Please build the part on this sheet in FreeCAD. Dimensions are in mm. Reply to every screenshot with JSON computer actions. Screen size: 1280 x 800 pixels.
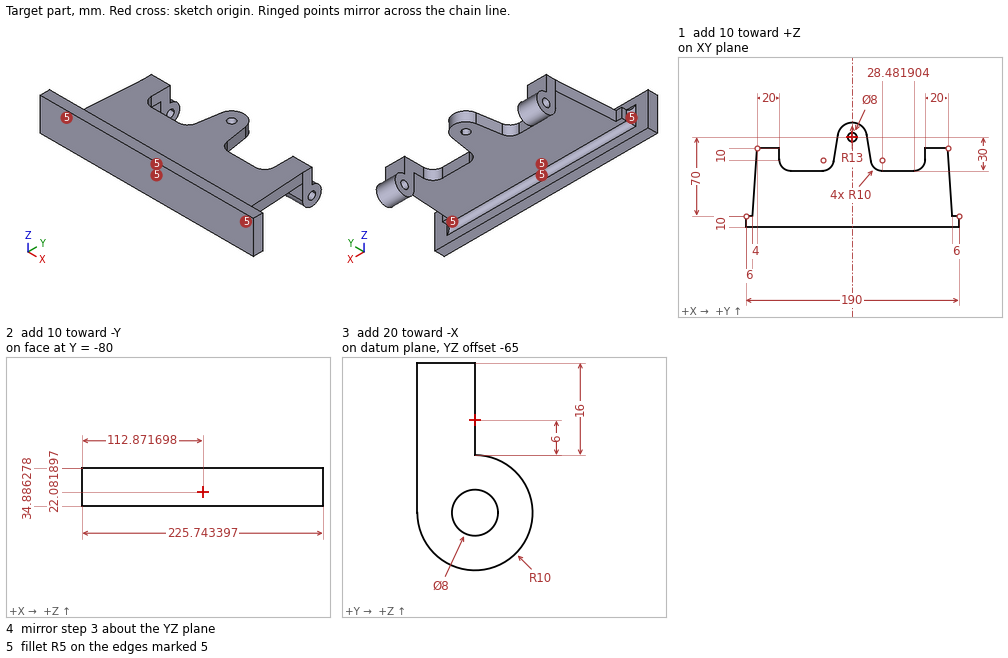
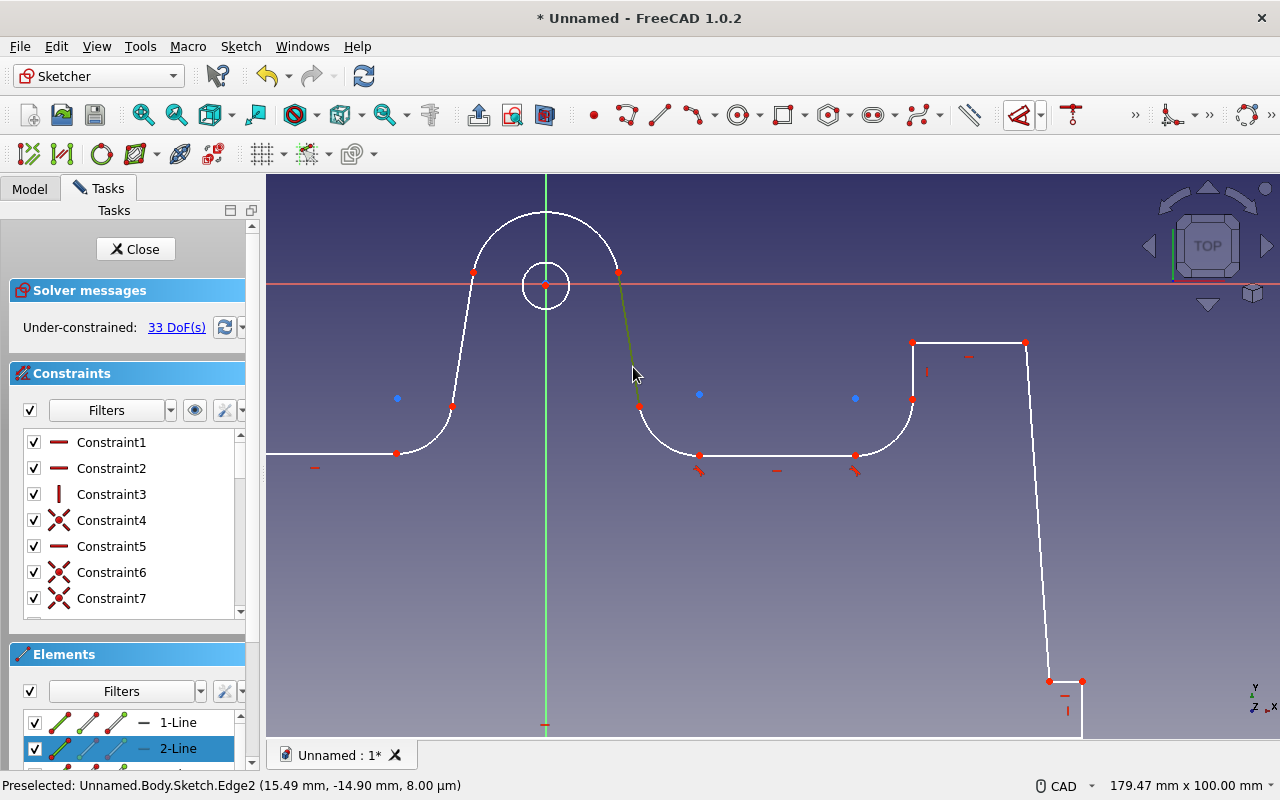
{"action": "left_click", "coordinate": [649, 430]}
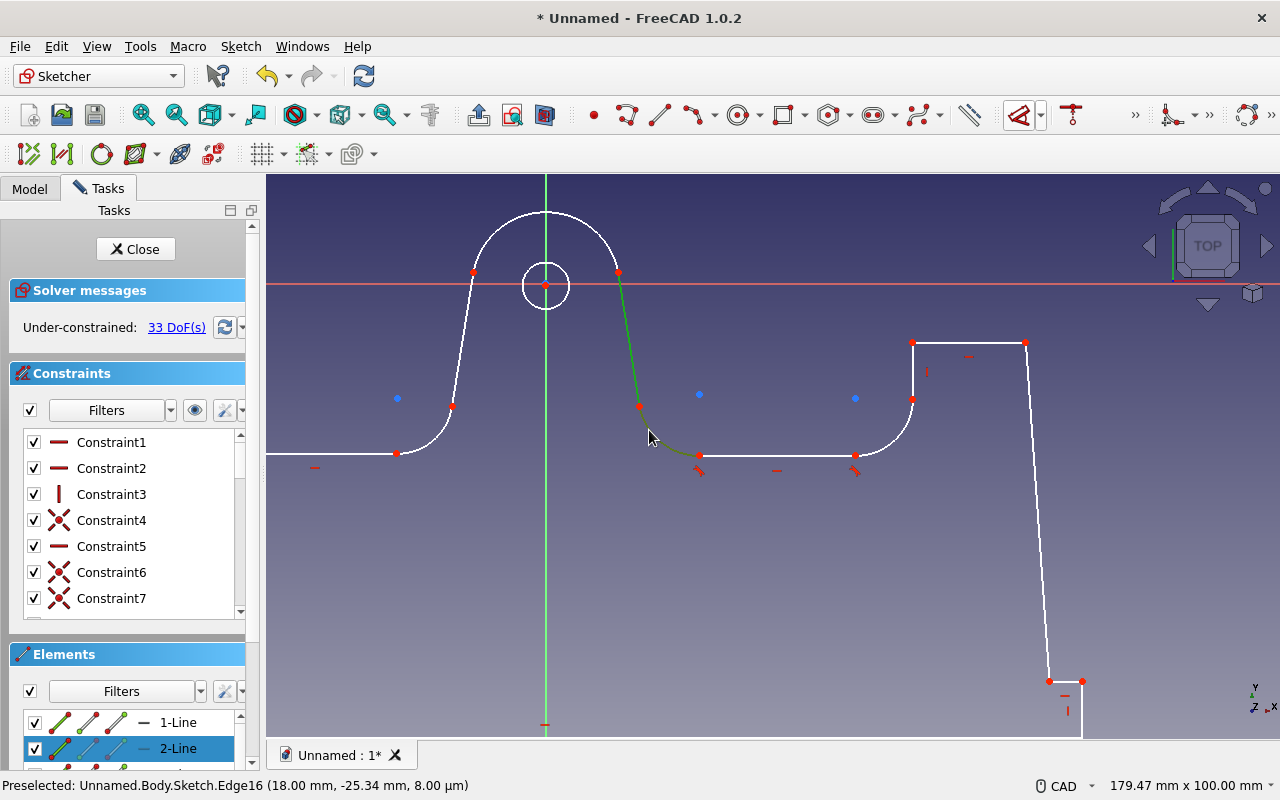
{"action": "key", "text": "t"}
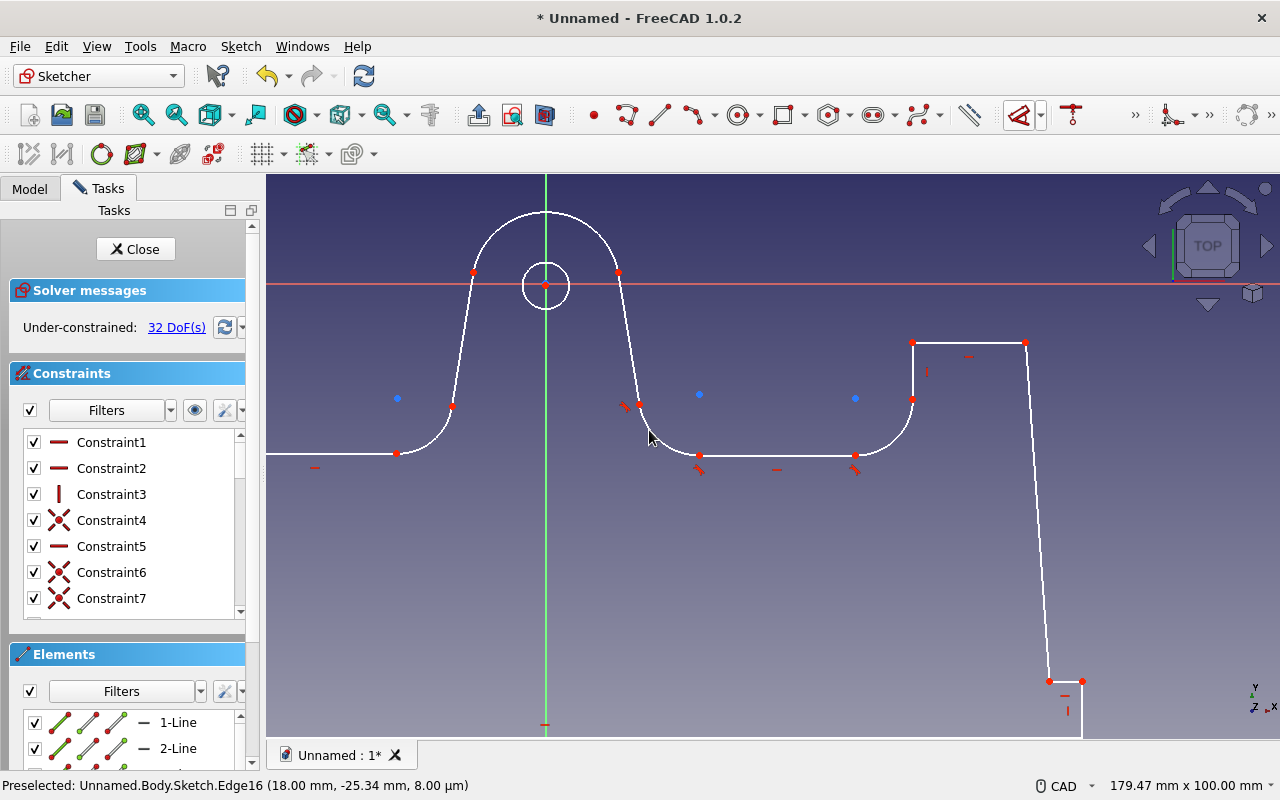
{"action": "left_click", "coordinate": [633, 365]}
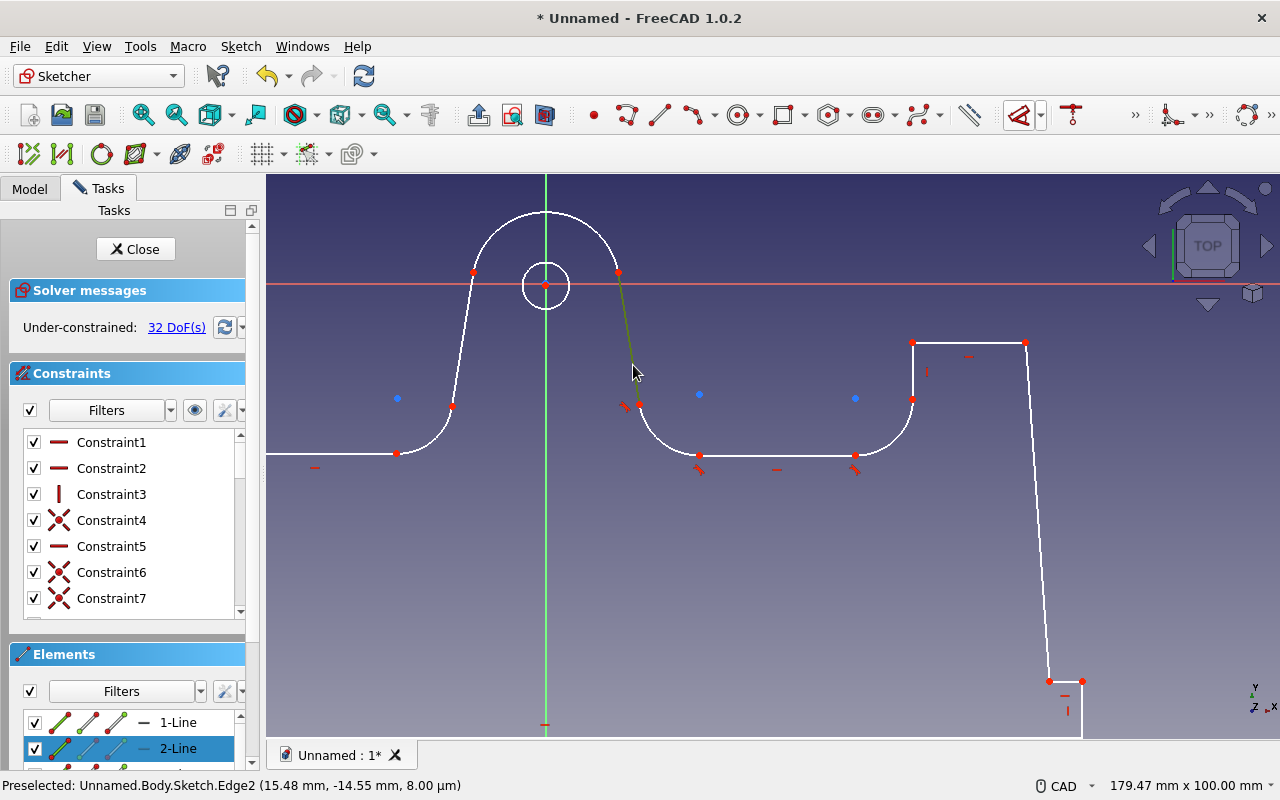
{"action": "left_click", "coordinate": [585, 223]}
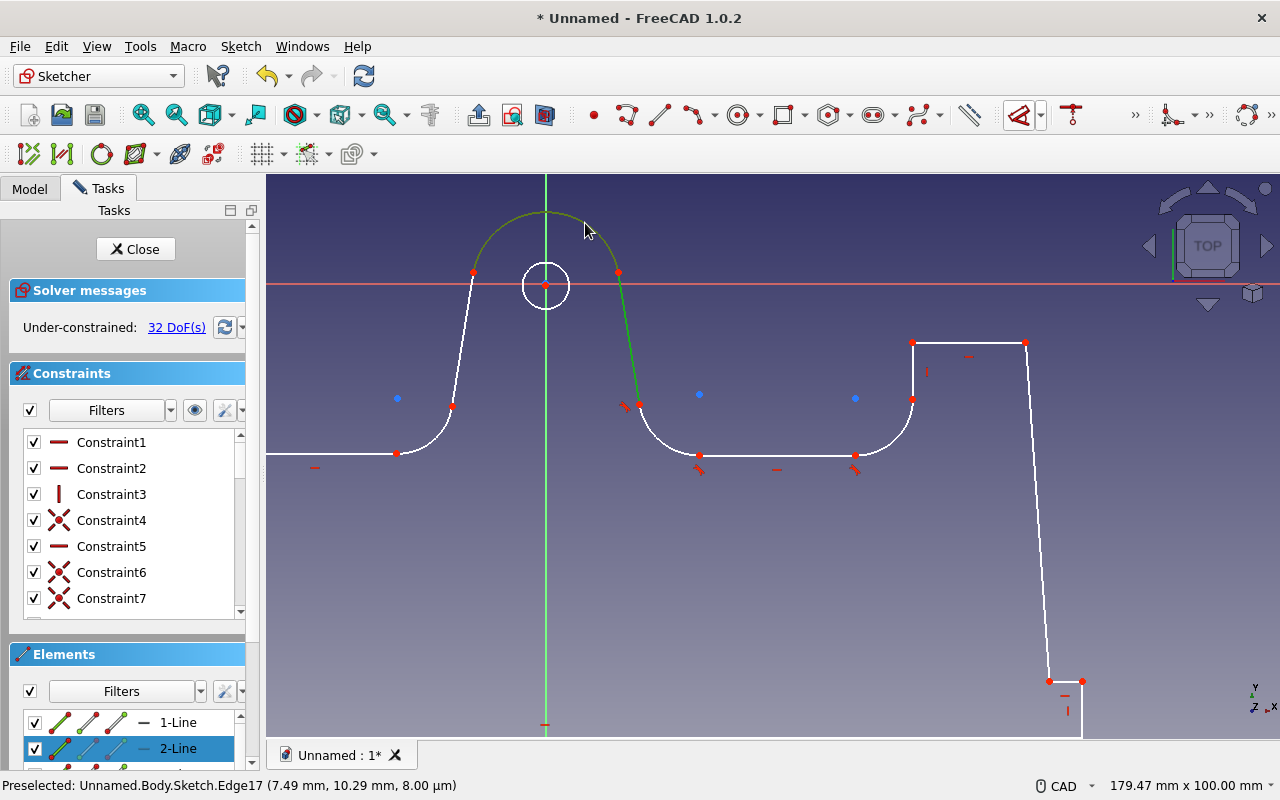
{"action": "key", "text": "t"}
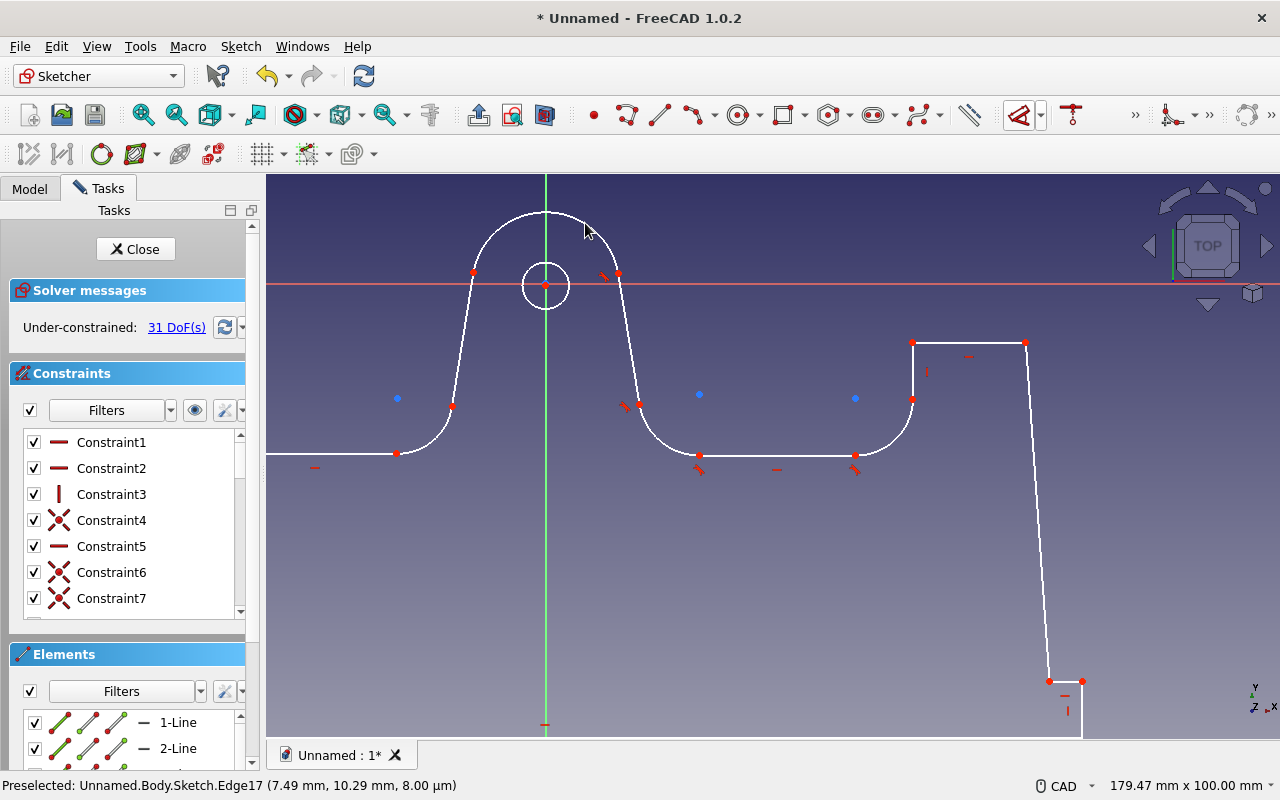
{"action": "left_click", "coordinate": [467, 313]}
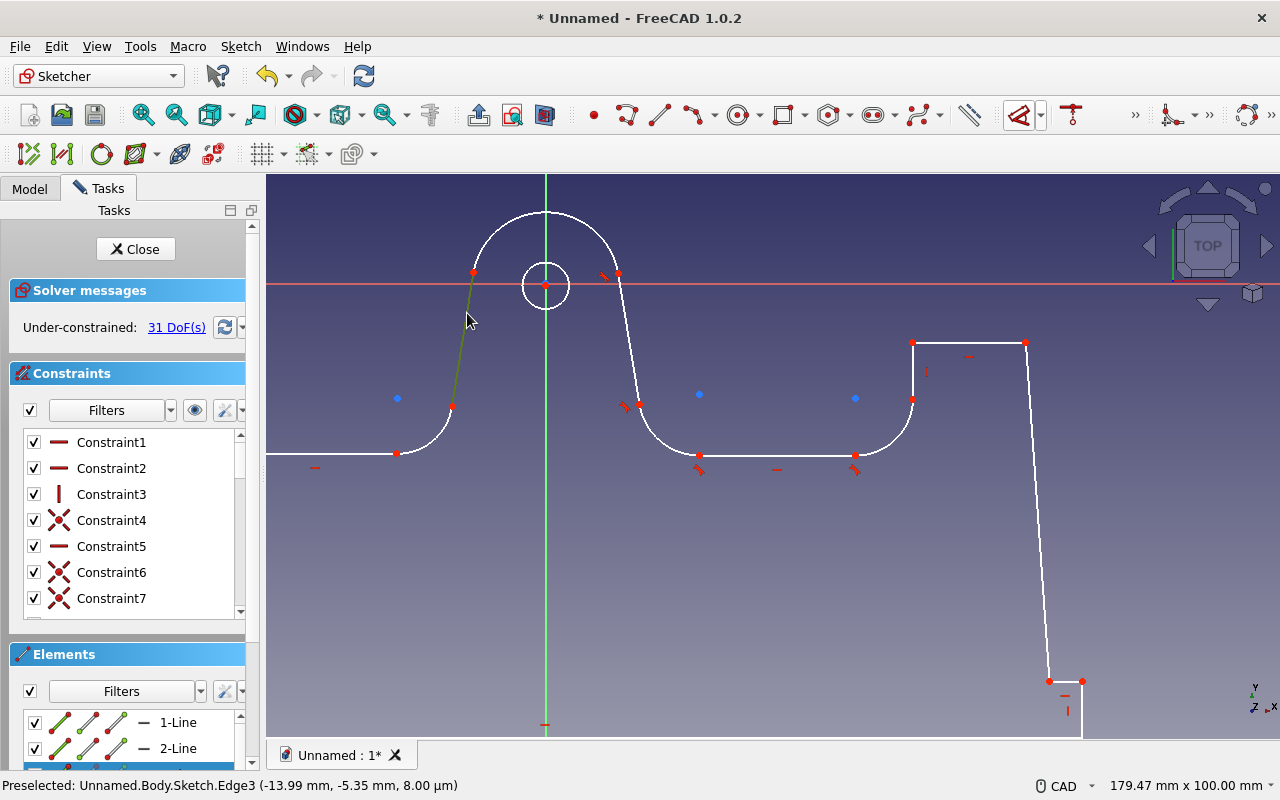
{"action": "left_click", "coordinate": [585, 224]}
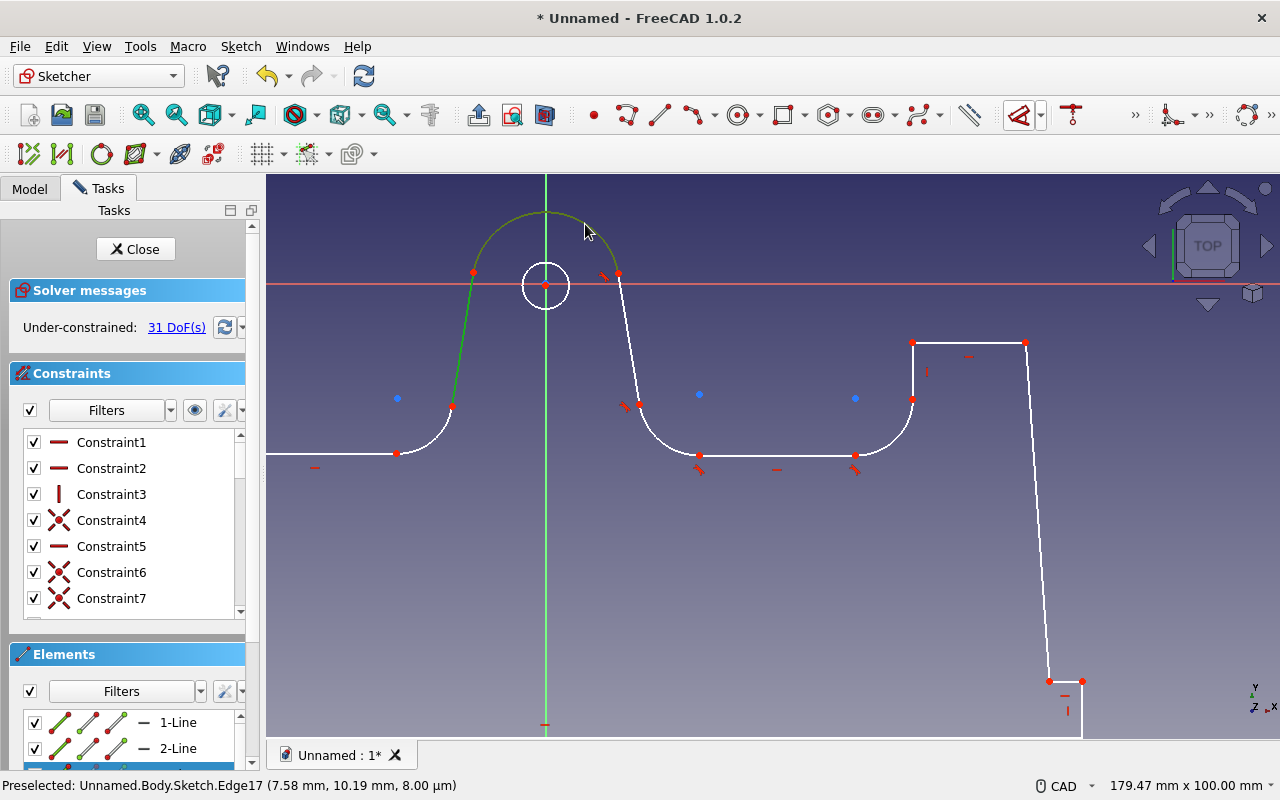
{"action": "key", "text": "t"}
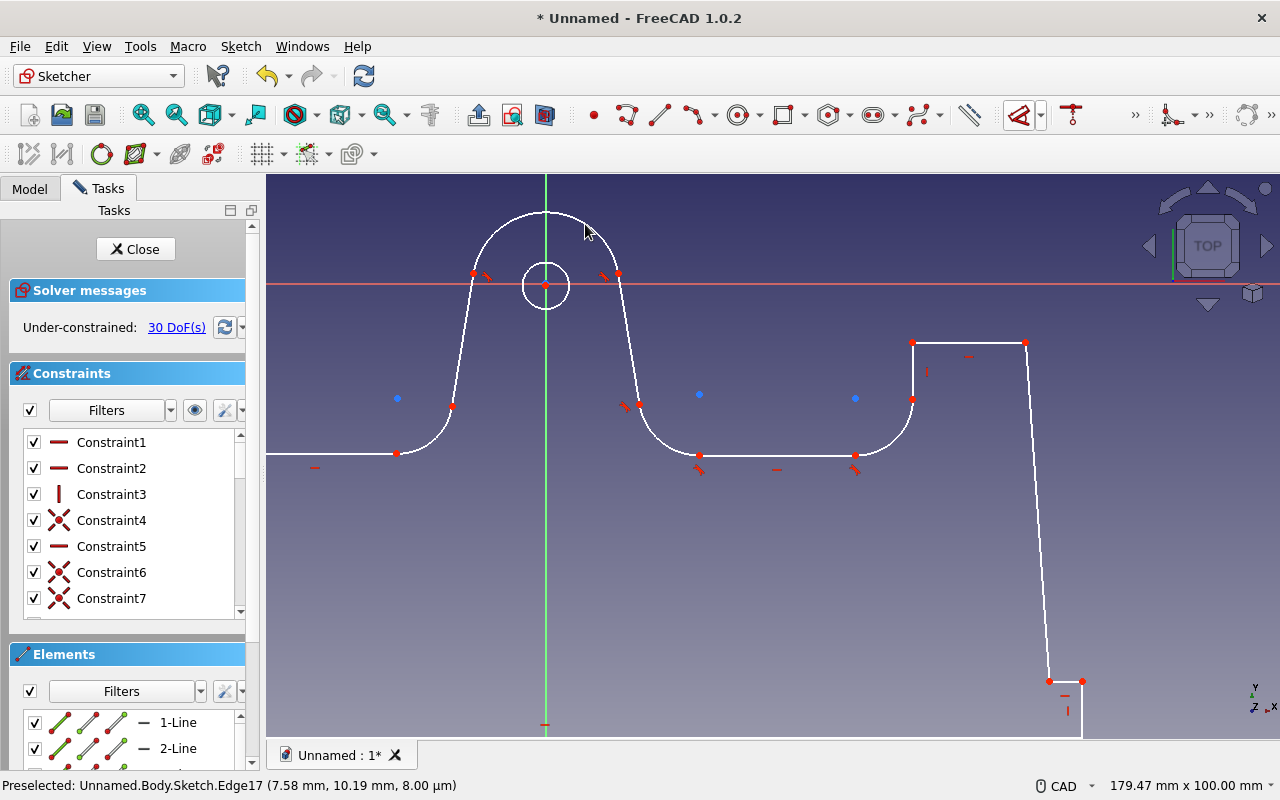
{"action": "left_click", "coordinate": [467, 314]}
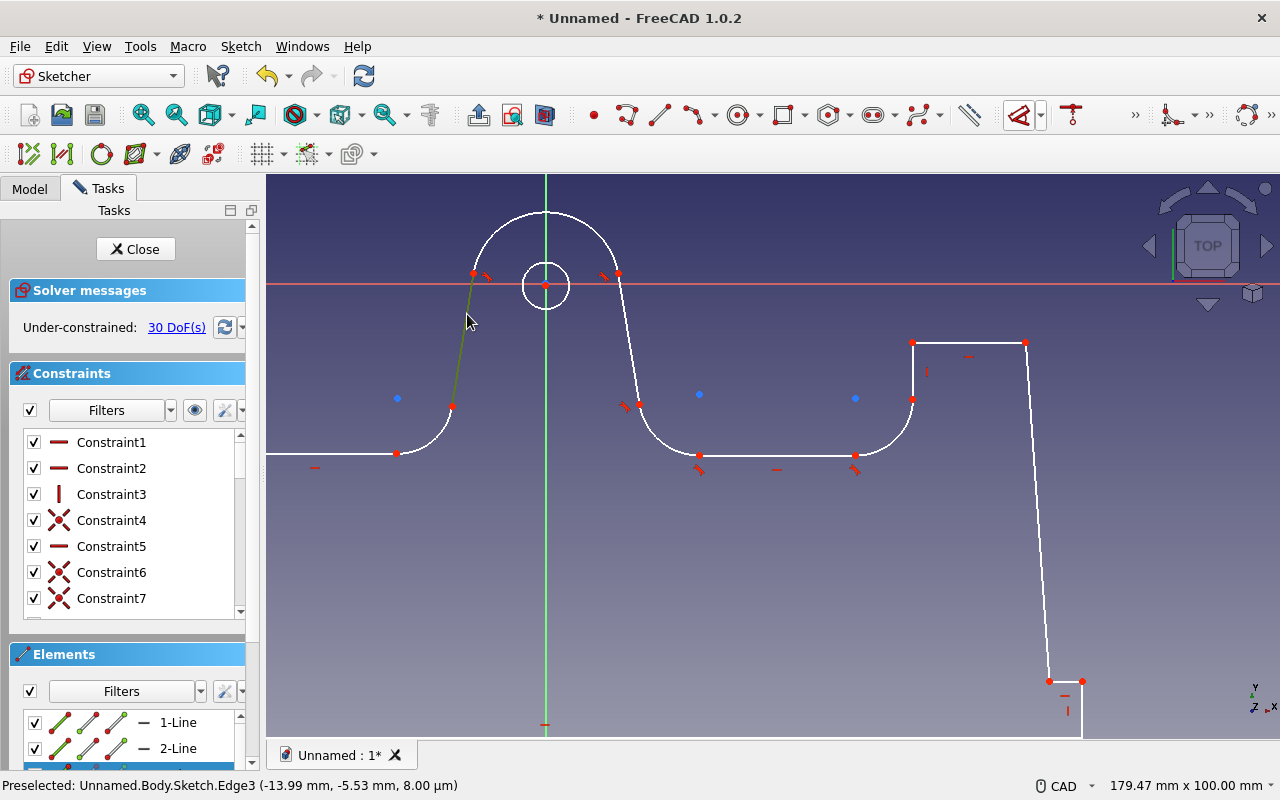
{"action": "left_click", "coordinate": [420, 449]}